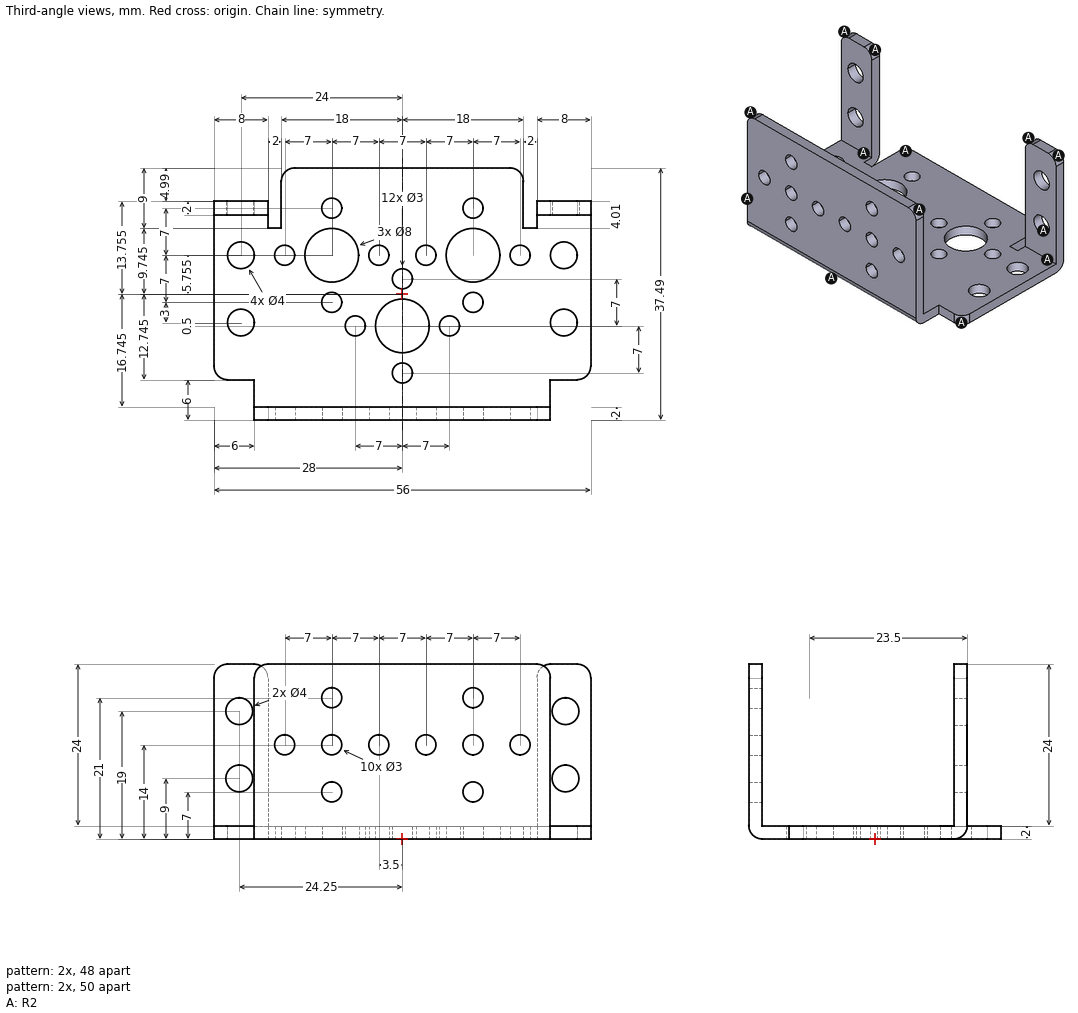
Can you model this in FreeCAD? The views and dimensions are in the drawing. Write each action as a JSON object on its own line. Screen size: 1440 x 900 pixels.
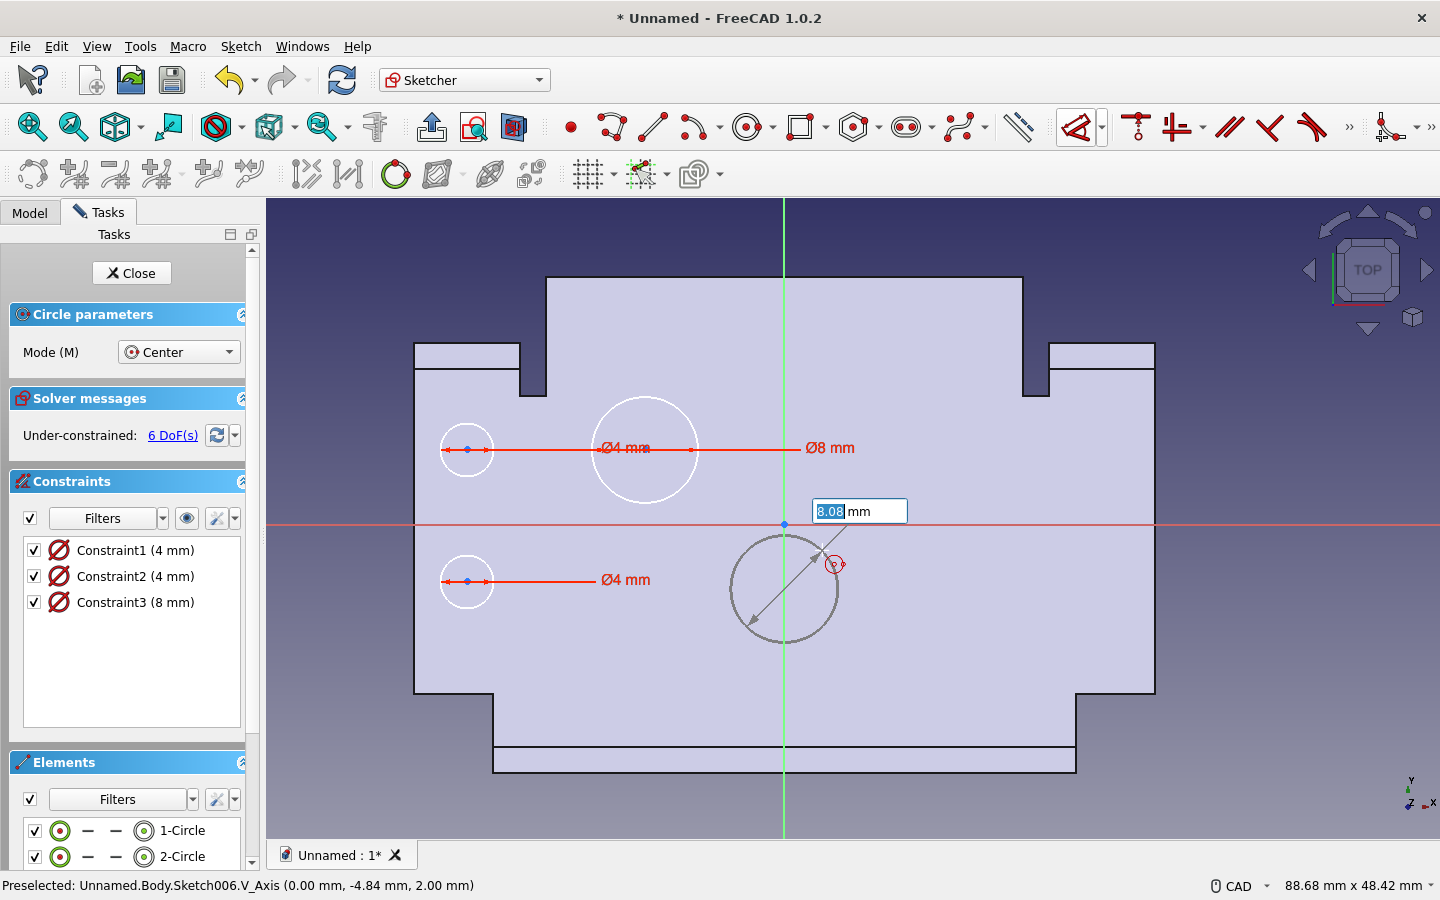
{"action": "type", "text": "8"}
{"action": "key", "text": "Return"}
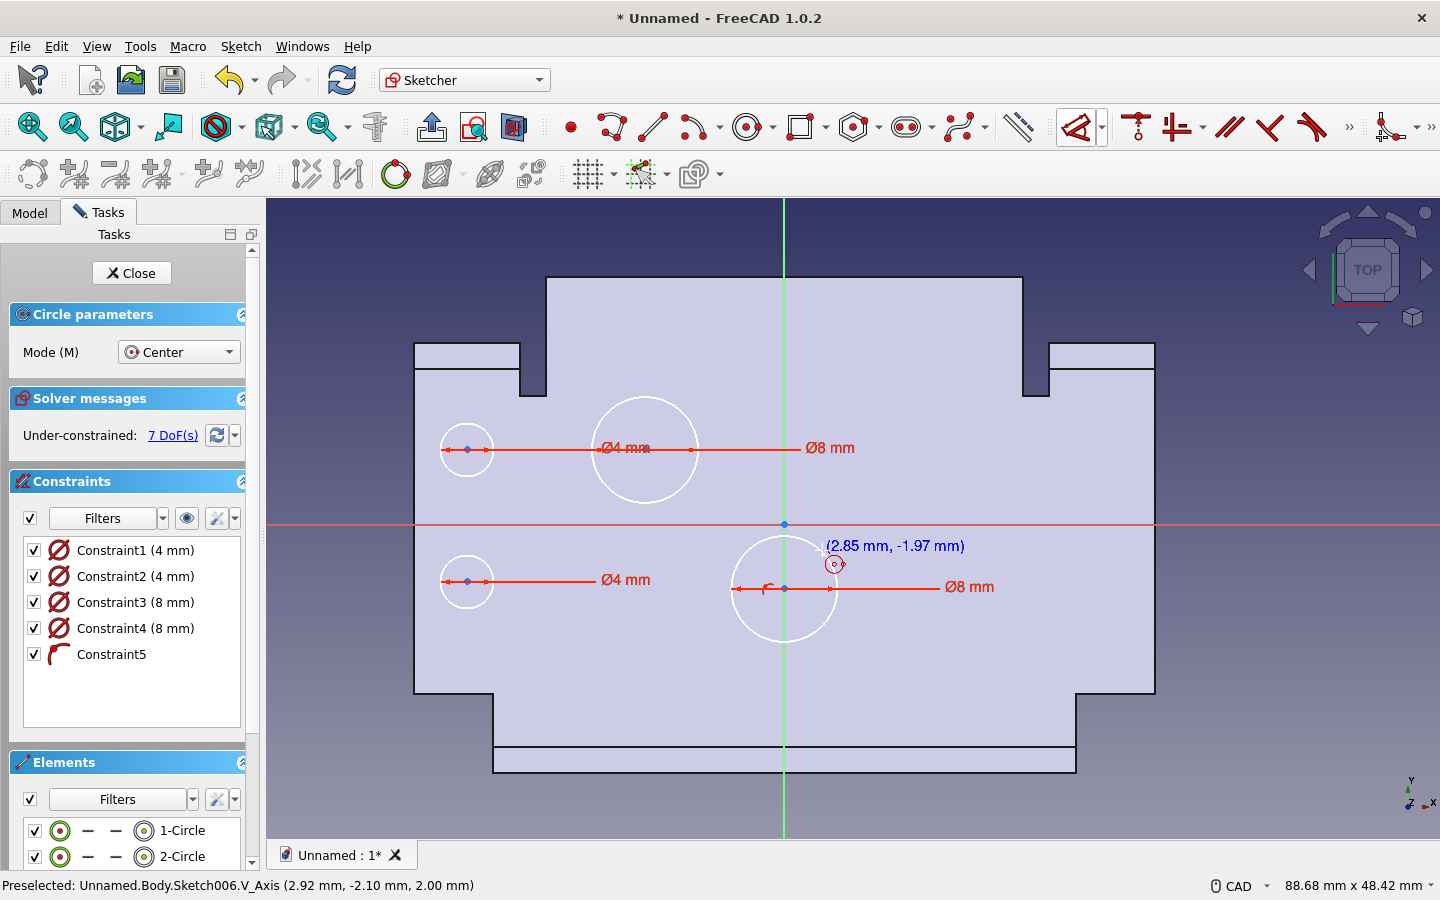
{"action": "left_click", "coordinate": [784, 495]}
{"action": "mouse_move", "coordinate": [798, 481]}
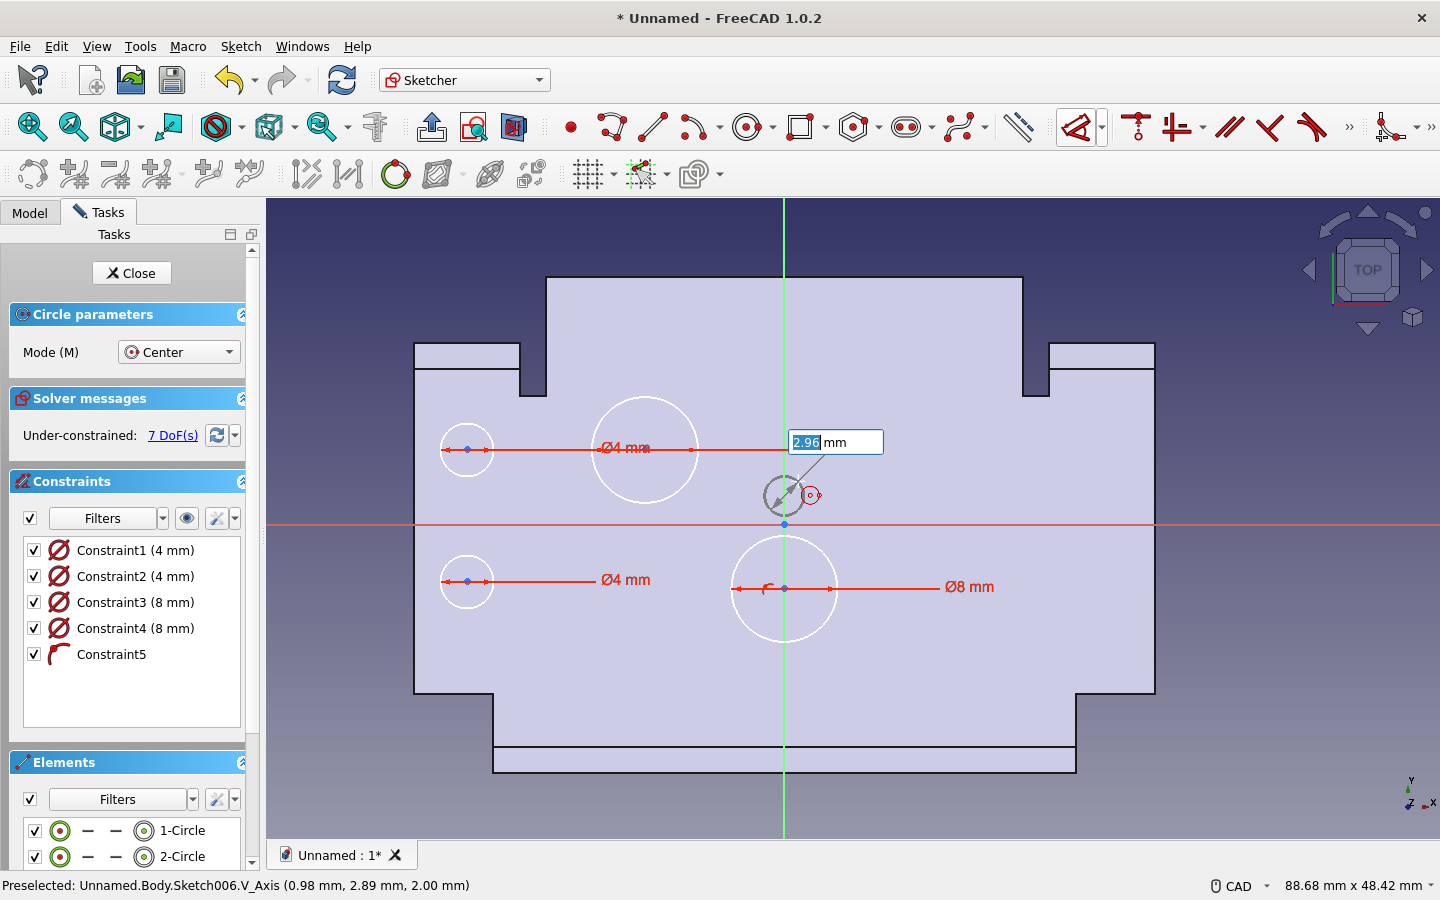
{"action": "type", "text": "3"}
{"action": "key", "text": "Return"}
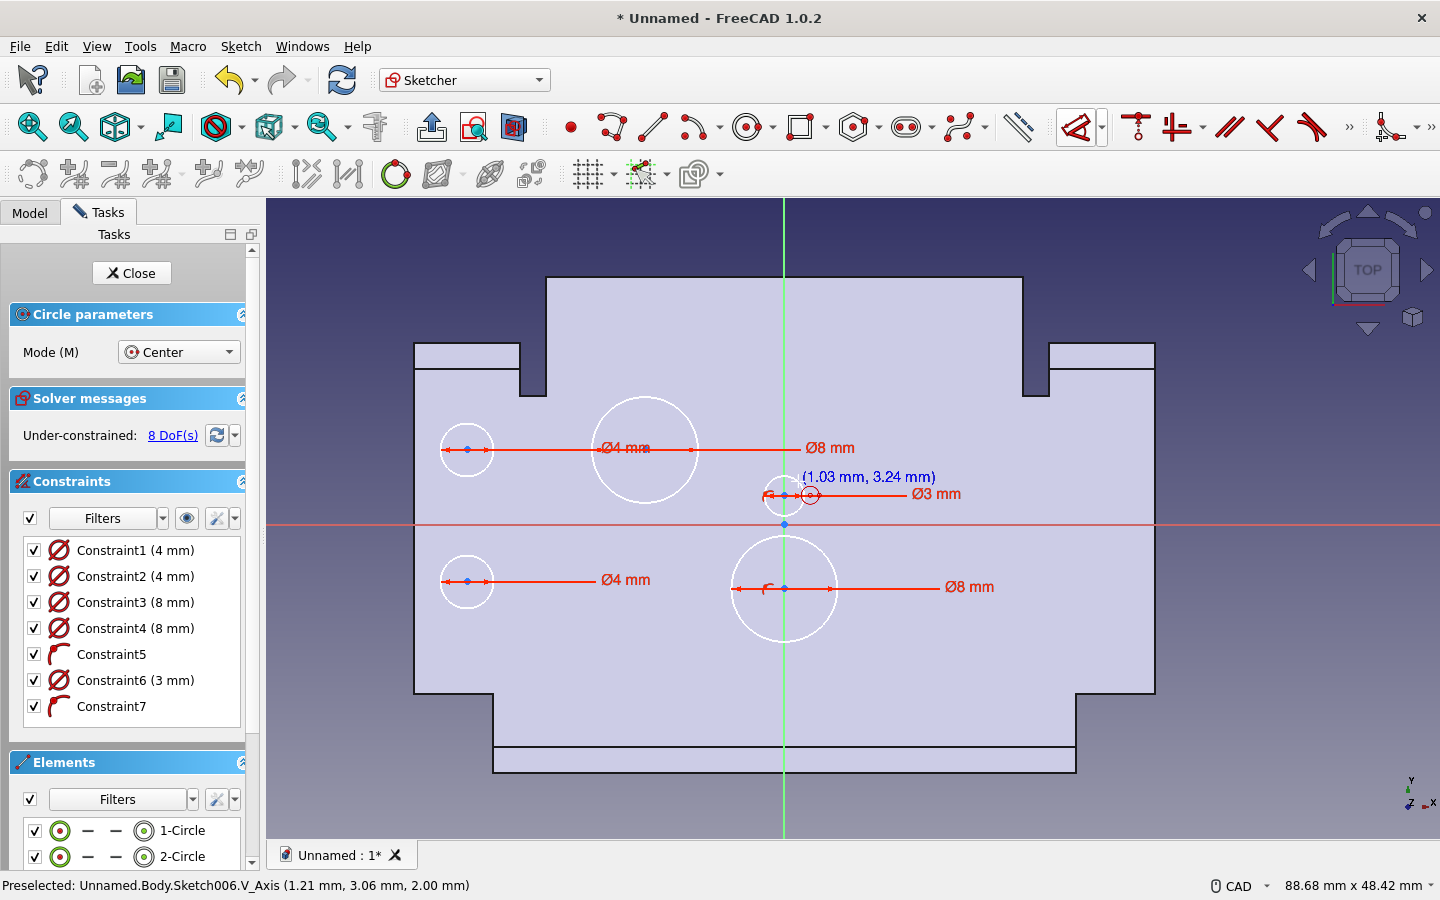
{"action": "left_click", "coordinate": [784, 680]}
{"action": "mouse_move", "coordinate": [798, 666]}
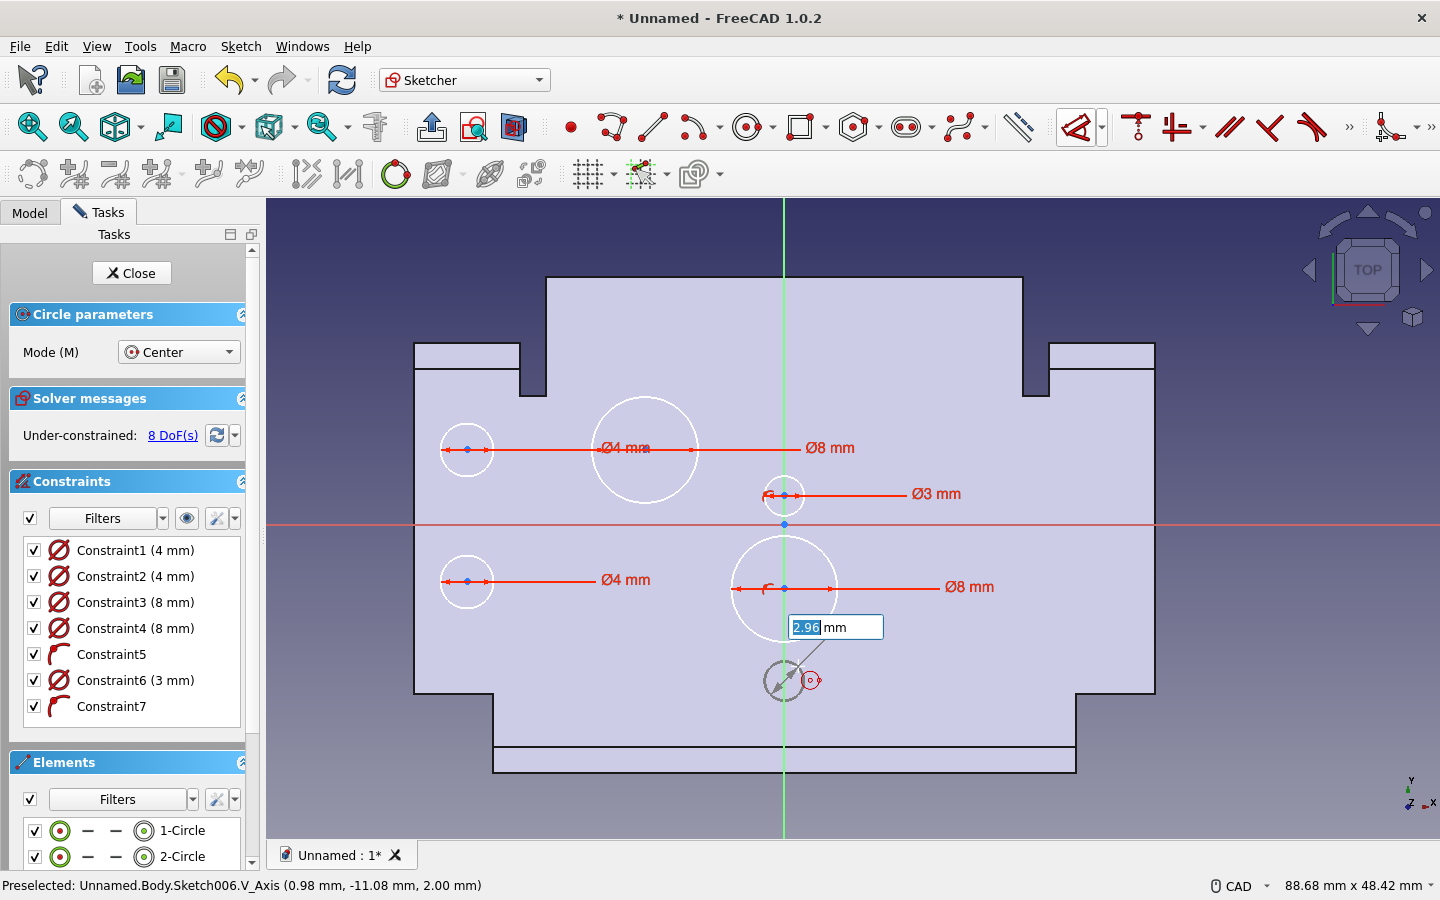
{"action": "type", "text": "3"}
{"action": "key", "text": "Return"}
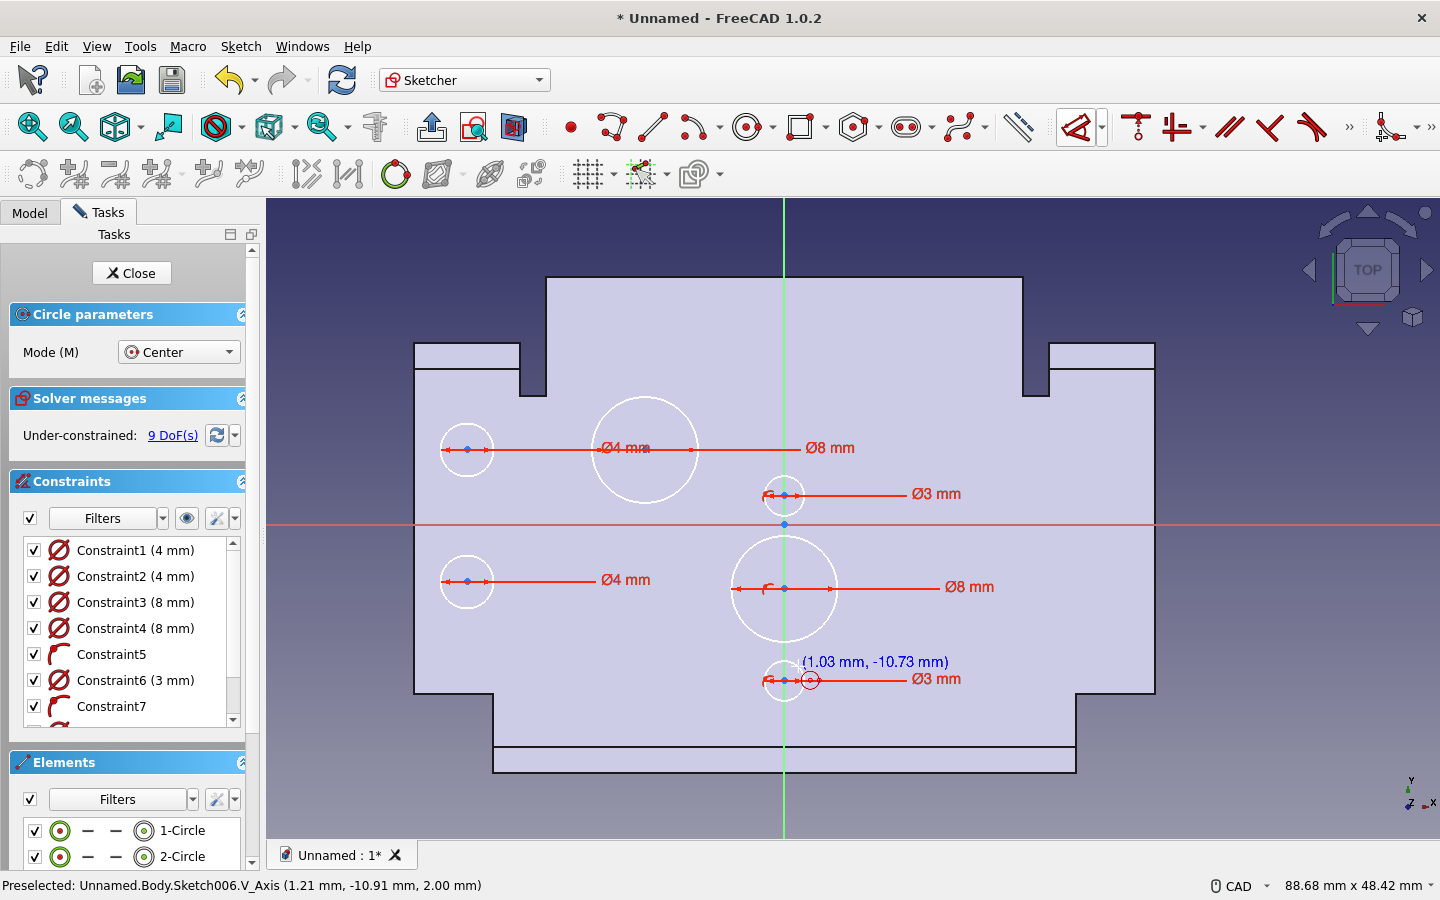
{"action": "left_click", "coordinate": [645, 541]}
{"action": "mouse_move", "coordinate": [659, 555]}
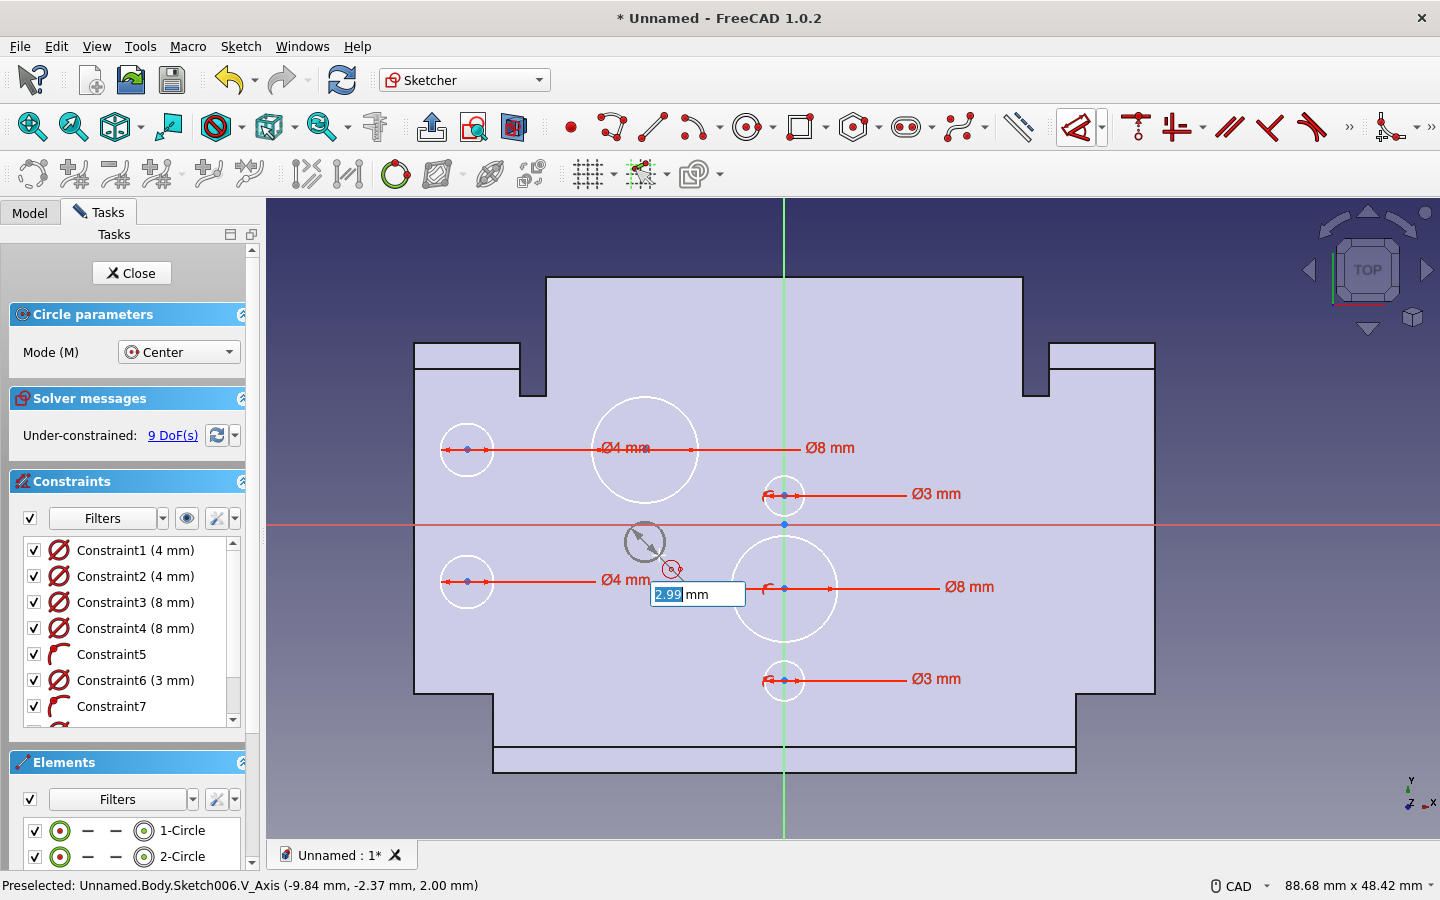
{"action": "type", "text": "3"}
{"action": "key", "text": "Return"}